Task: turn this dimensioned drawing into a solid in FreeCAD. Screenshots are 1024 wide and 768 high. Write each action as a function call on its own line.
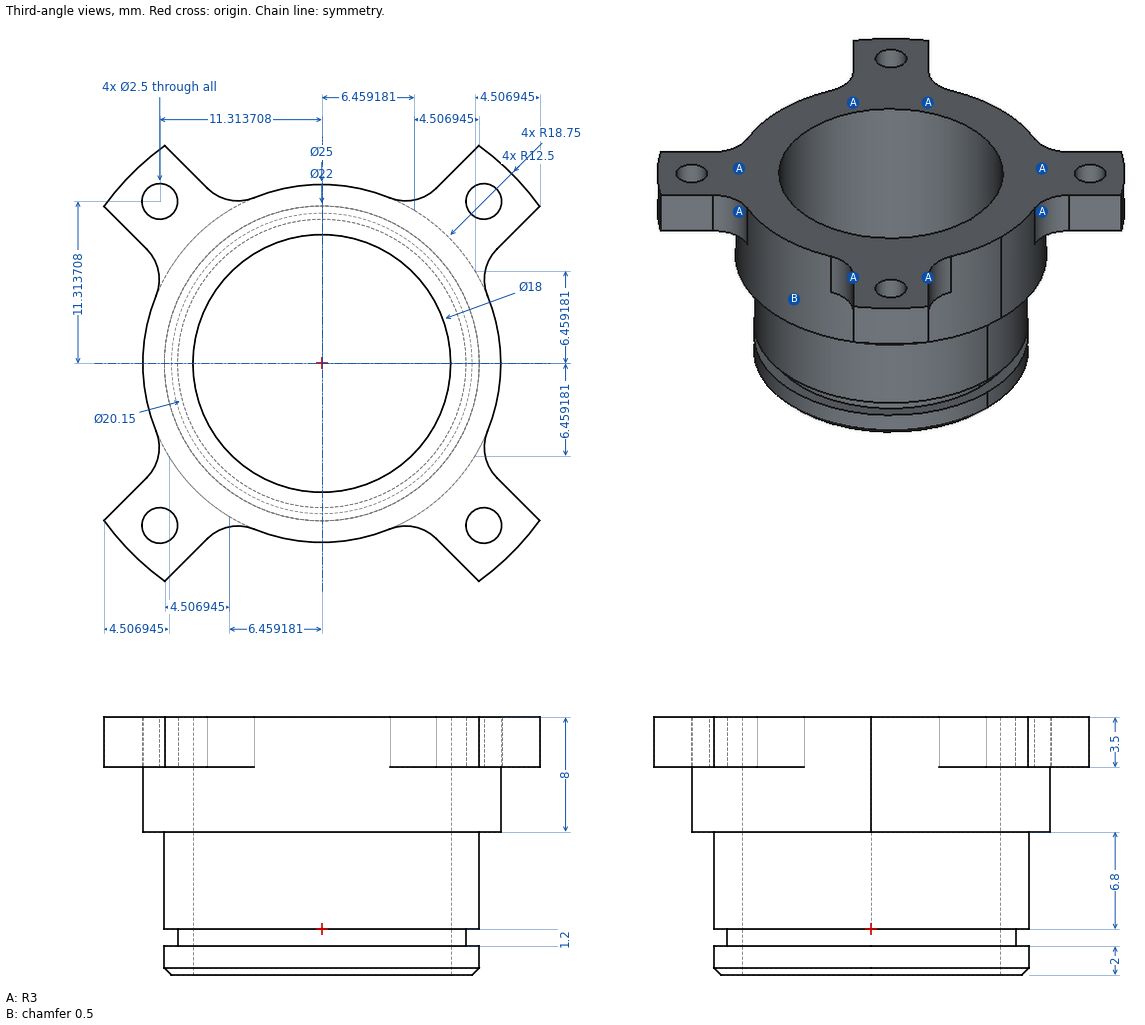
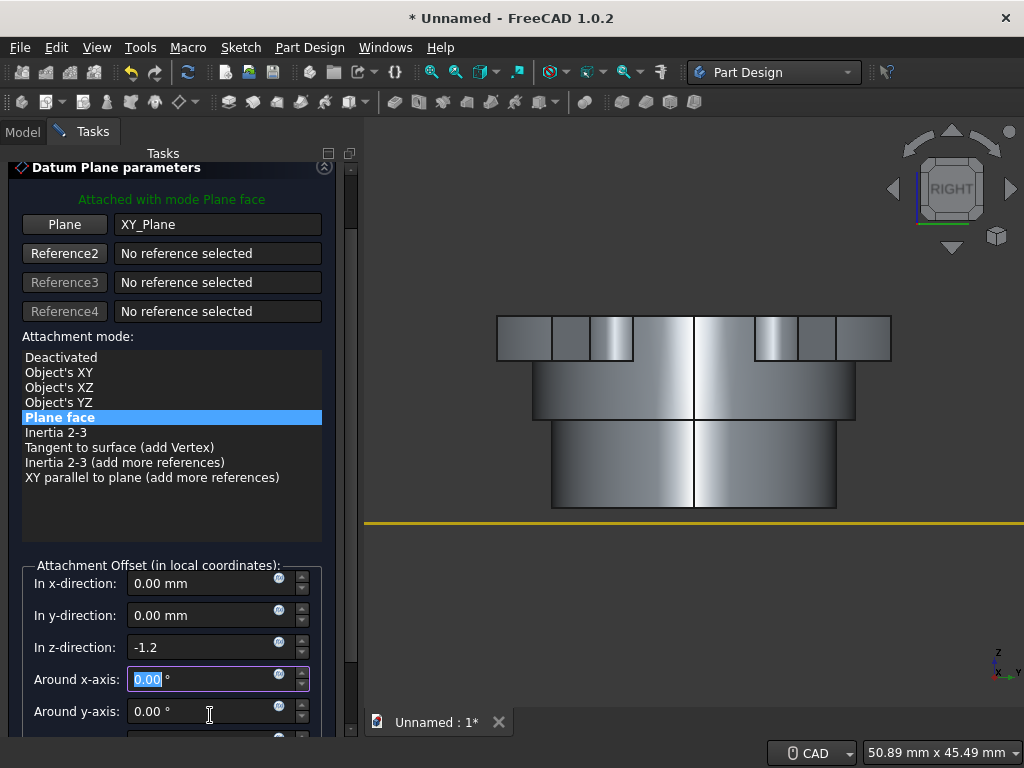
scroll(351, 450, up, 2)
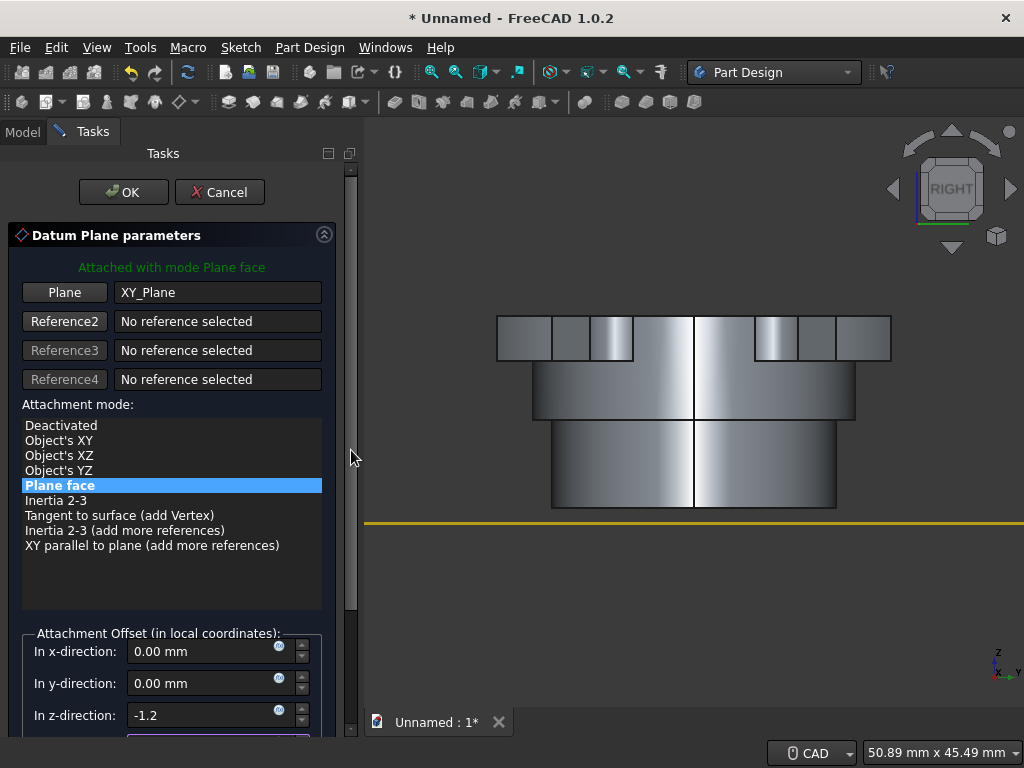
click(124, 192)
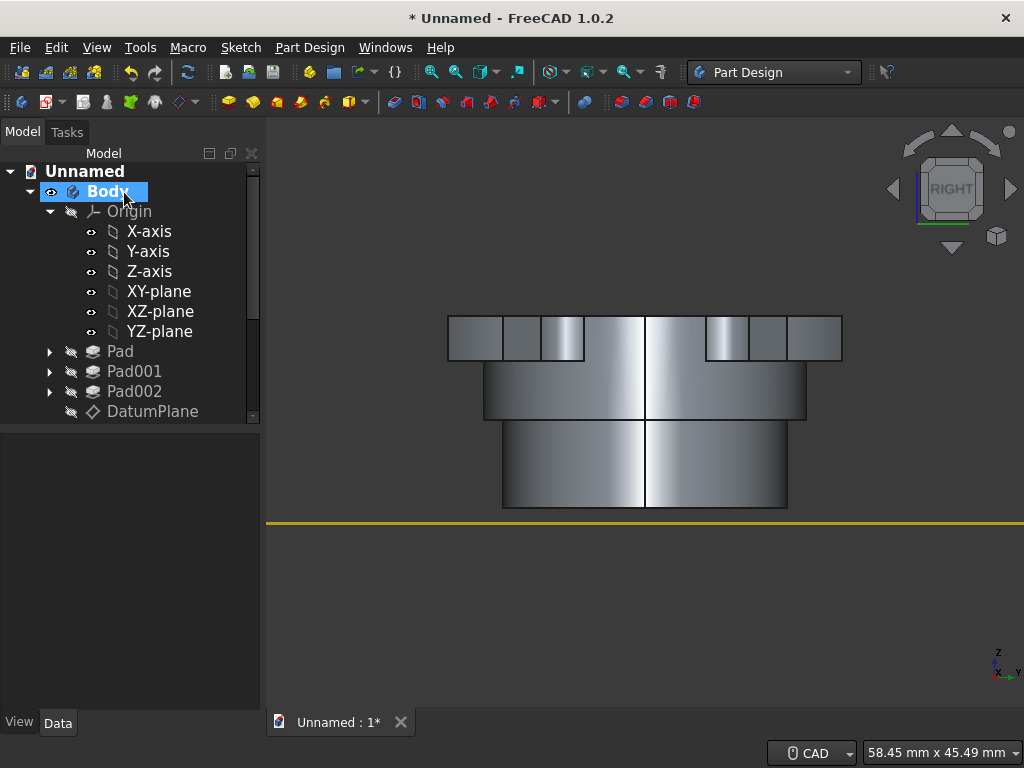
scroll(100, 287, down, 3)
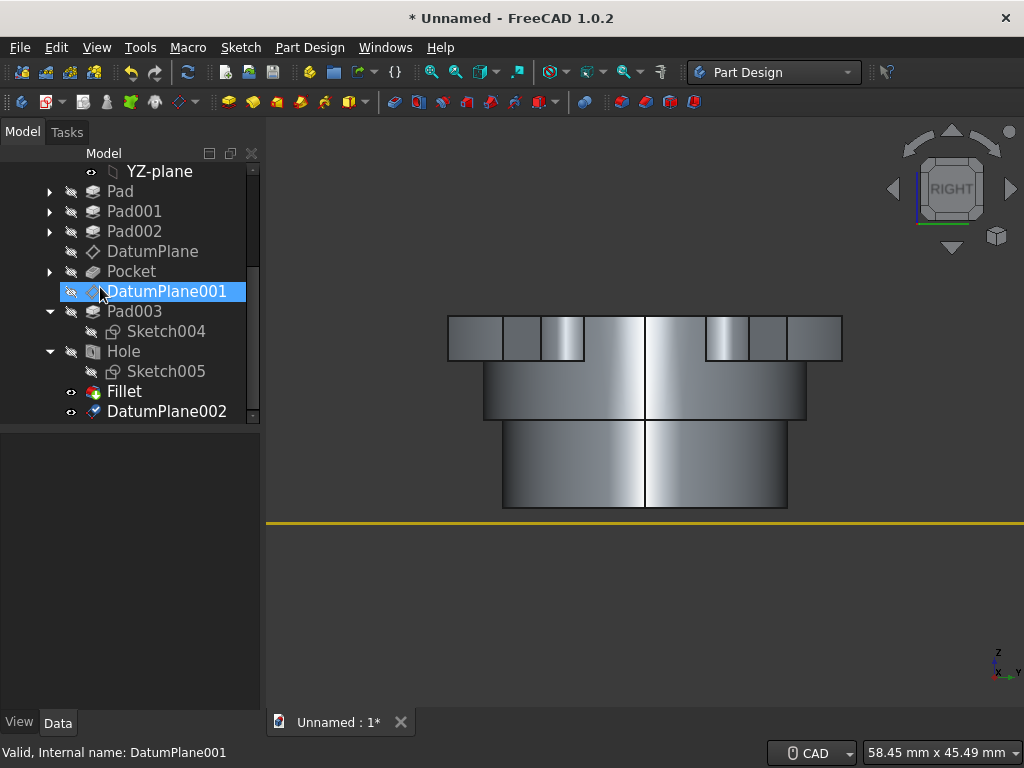
click(116, 412)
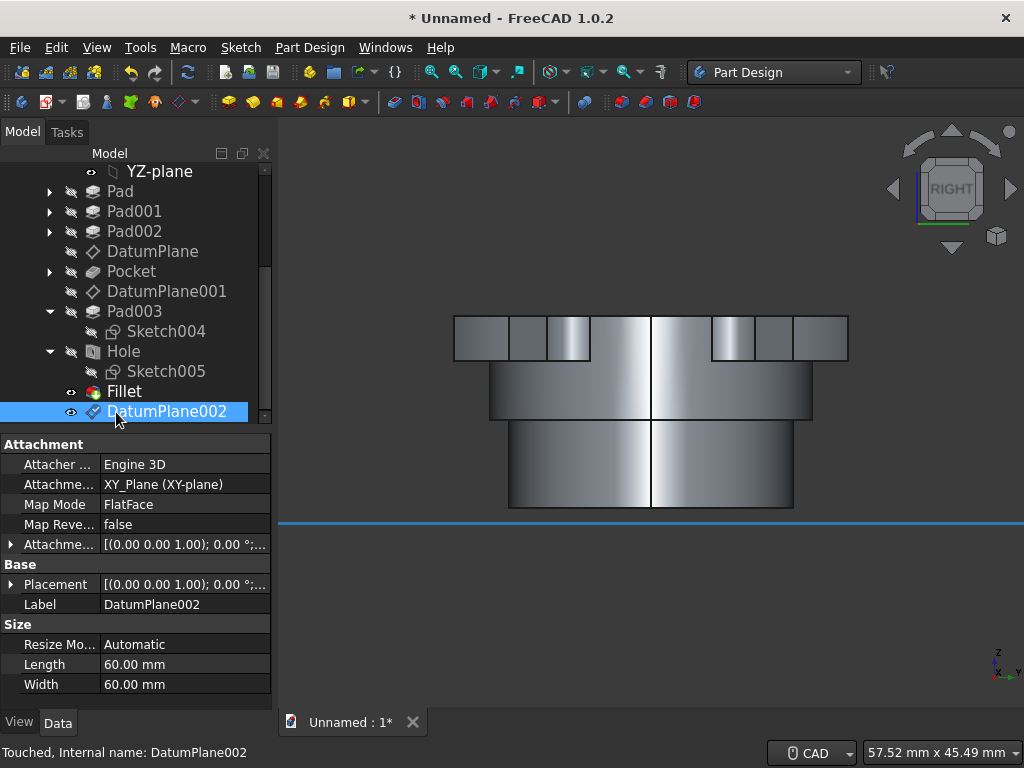
click(46, 102)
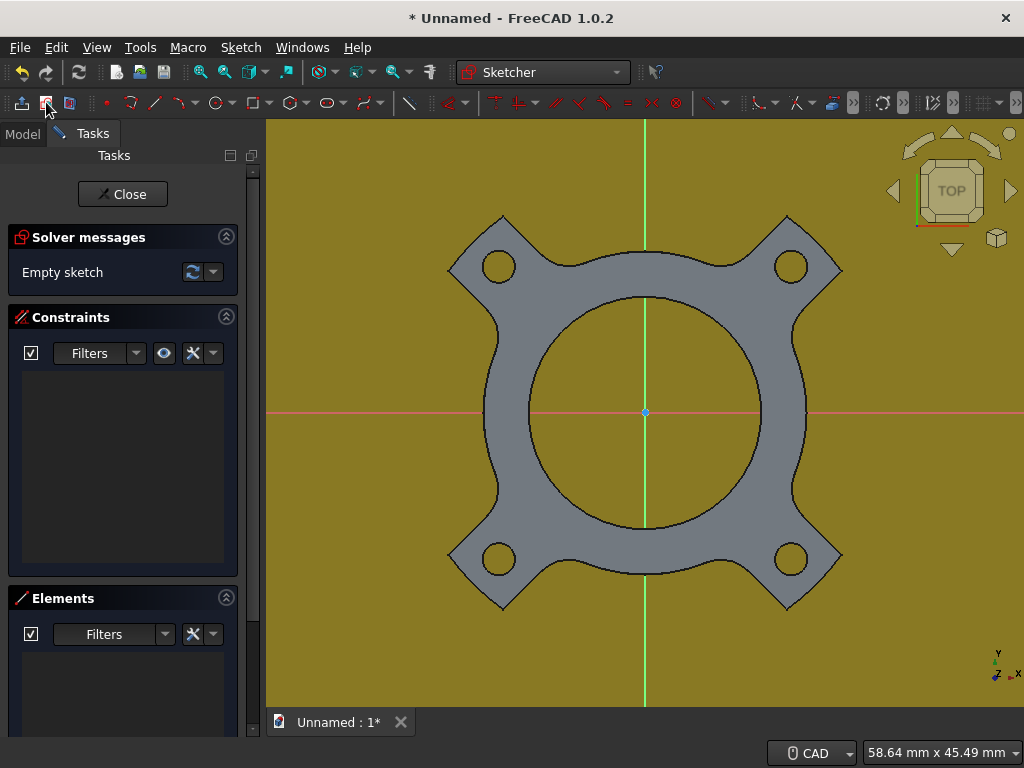
click(70, 104)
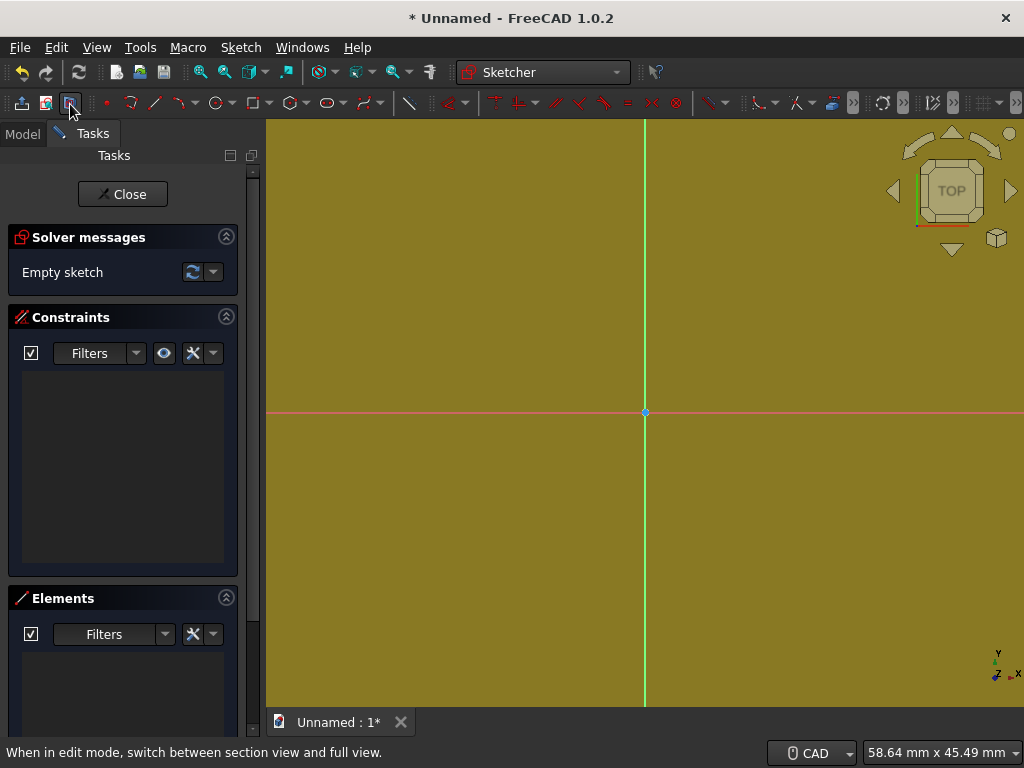
scroll(784, 413, up, 2)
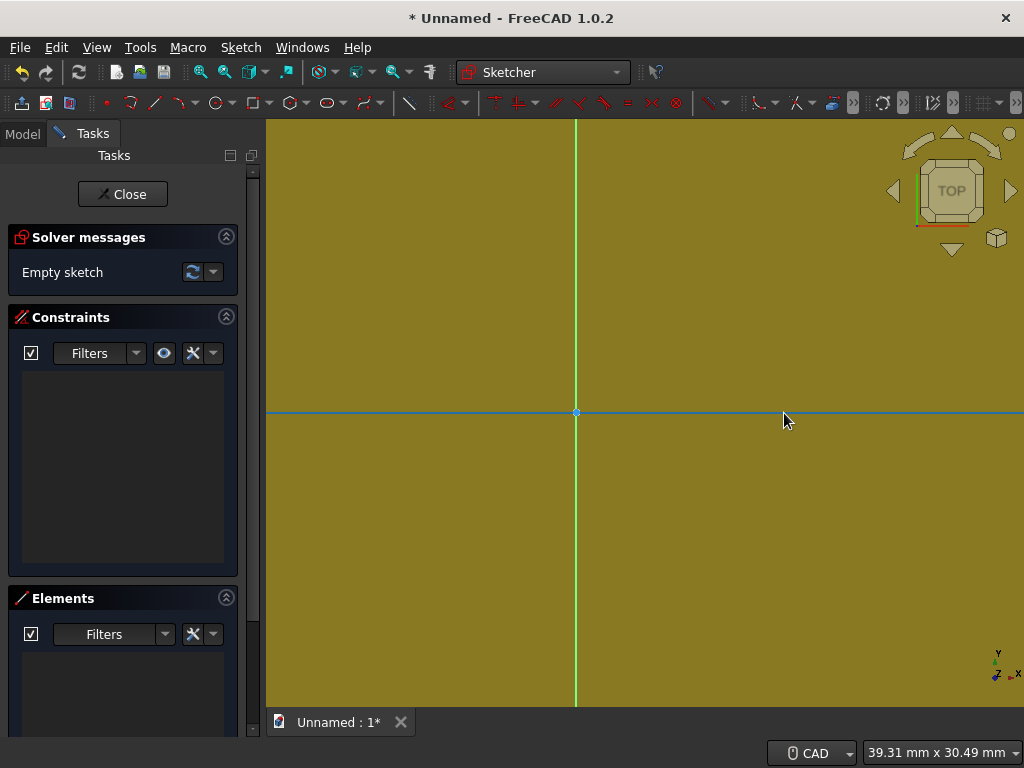
click(216, 104)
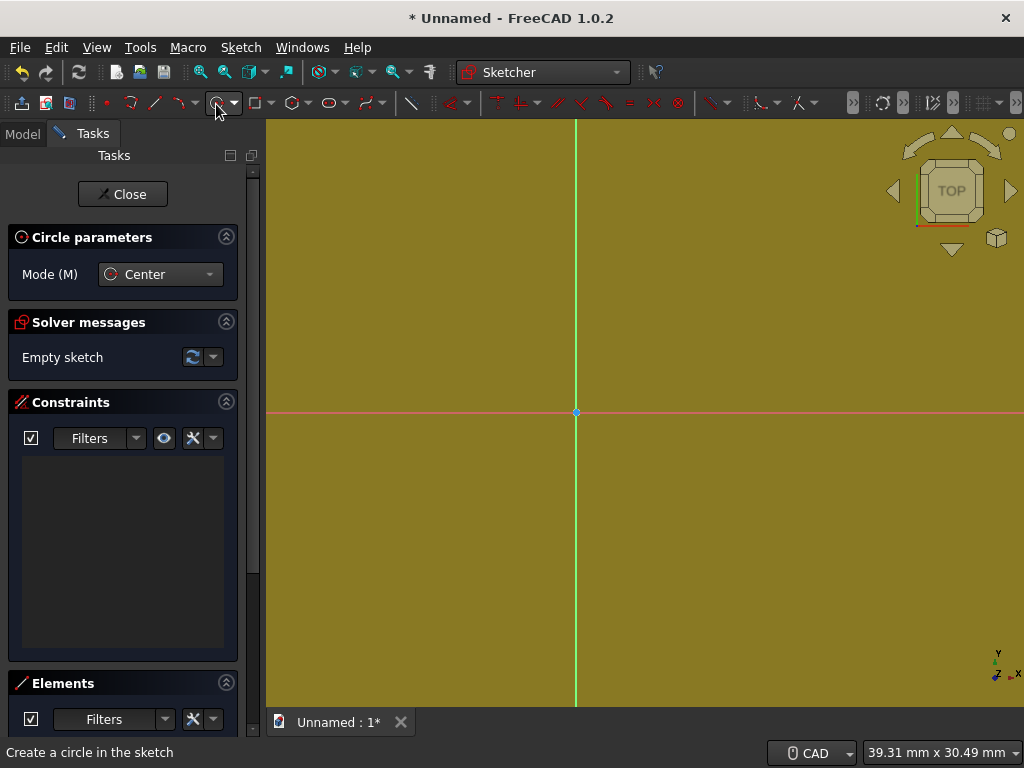
click(576, 413)
click(714, 275)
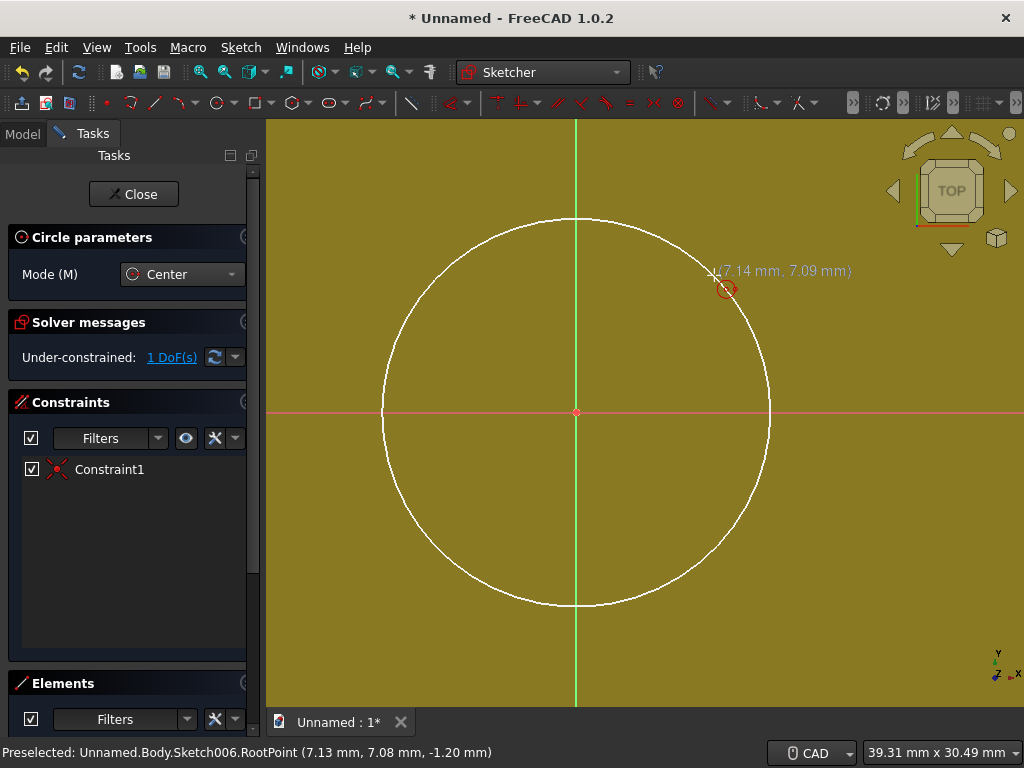
click(576, 413)
click(699, 290)
key(Escape)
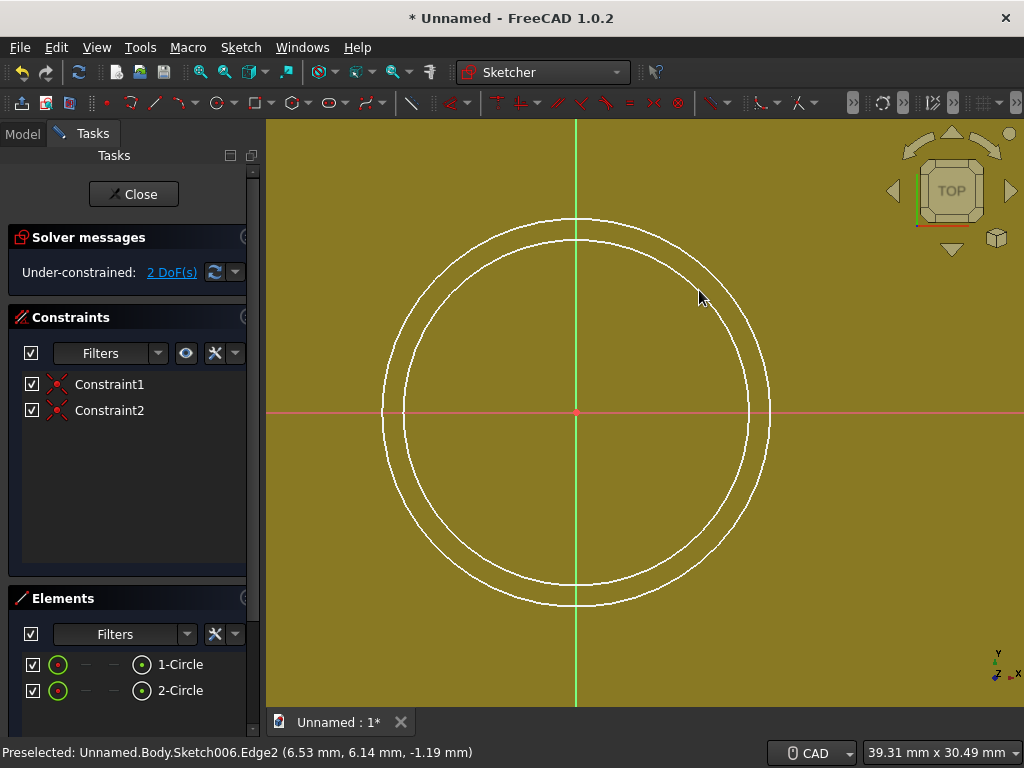
click(450, 104)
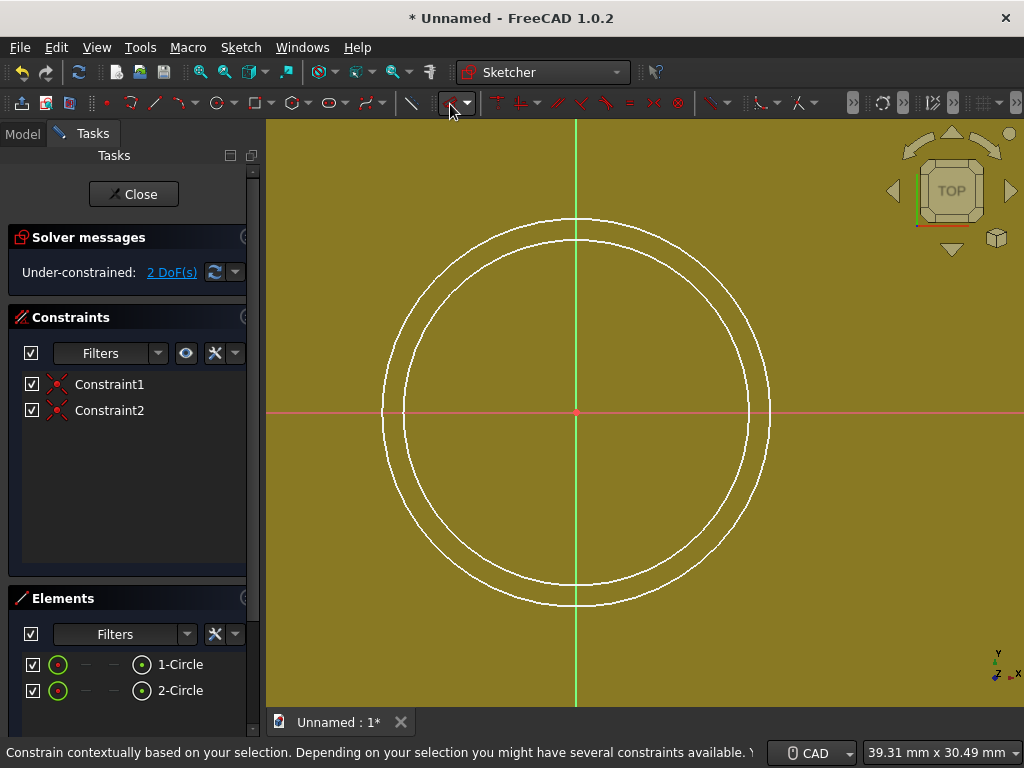
click(713, 275)
click(736, 252)